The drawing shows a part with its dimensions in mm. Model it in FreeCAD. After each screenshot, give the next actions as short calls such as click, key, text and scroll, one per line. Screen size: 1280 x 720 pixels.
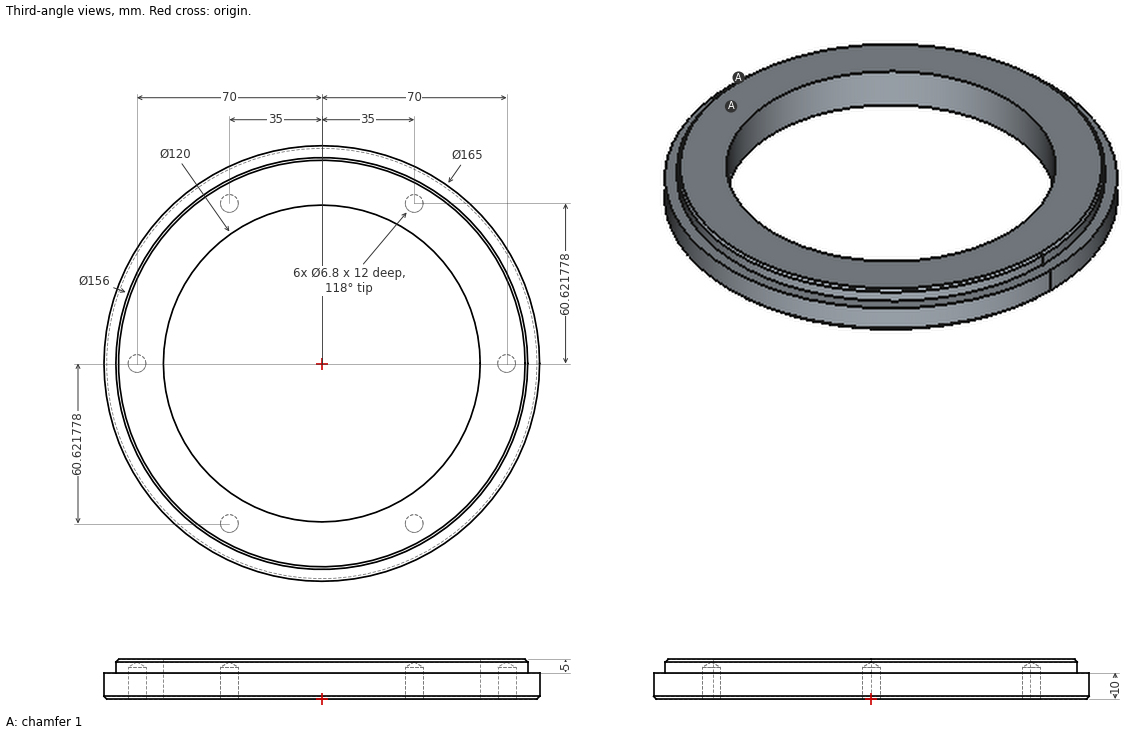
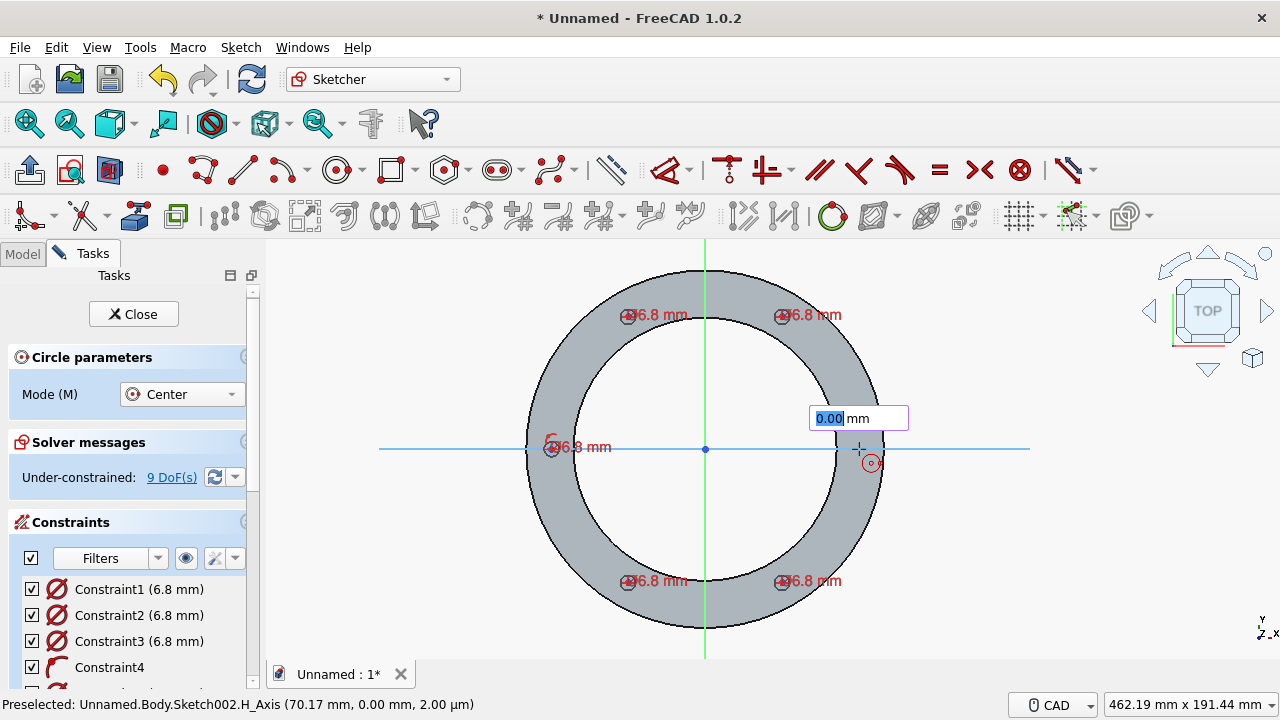
scroll(856, 456, up, 5)
move(855, 456)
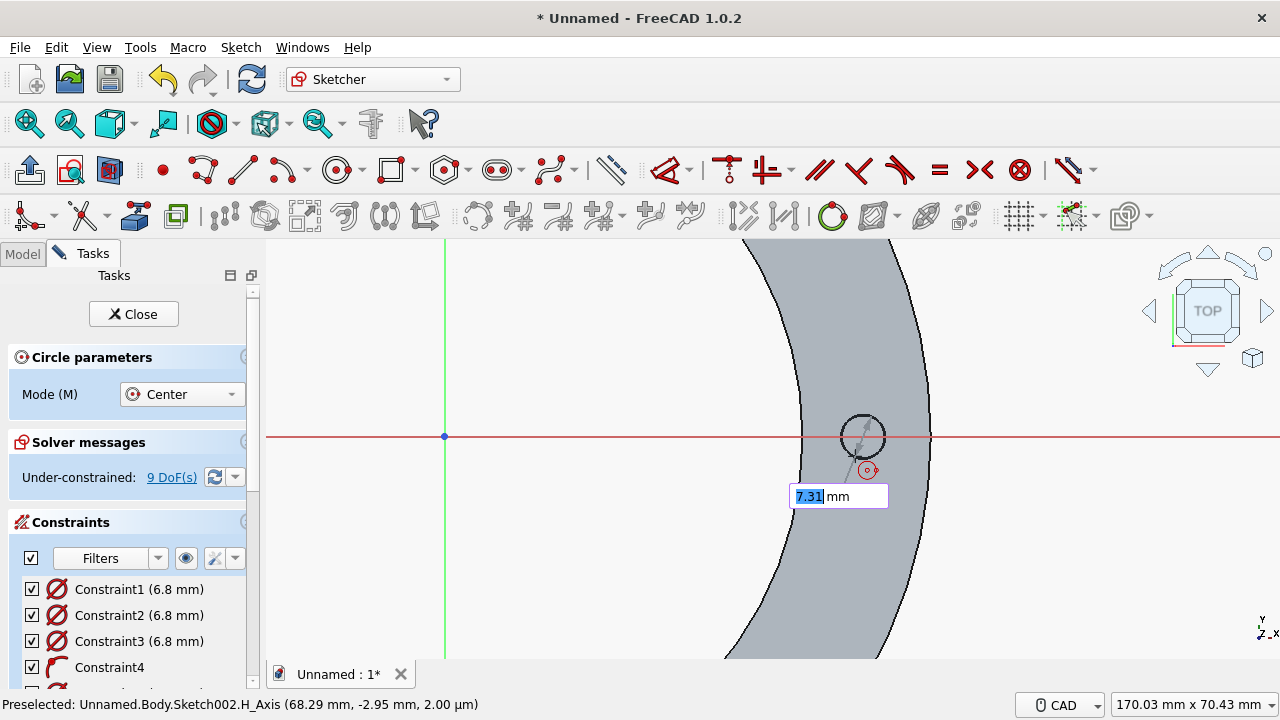
text(6.8)
key(Return)
key(Escape)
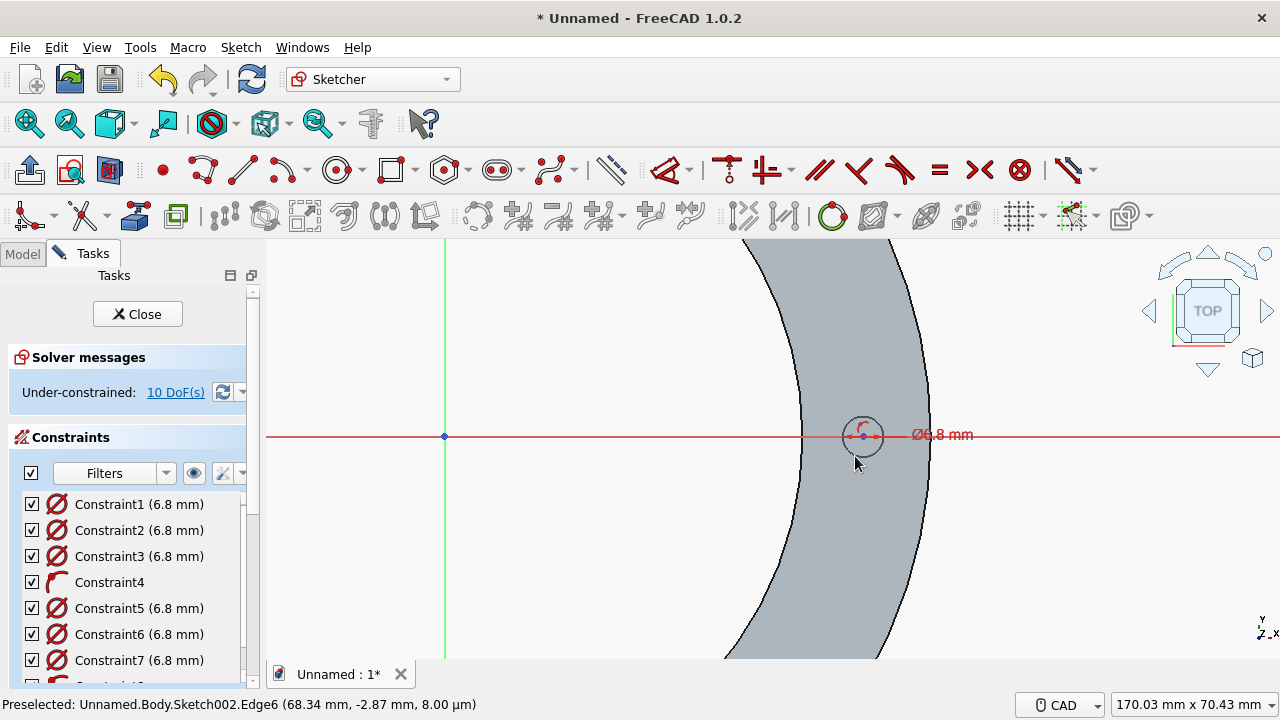
scroll(856, 456, down, 5)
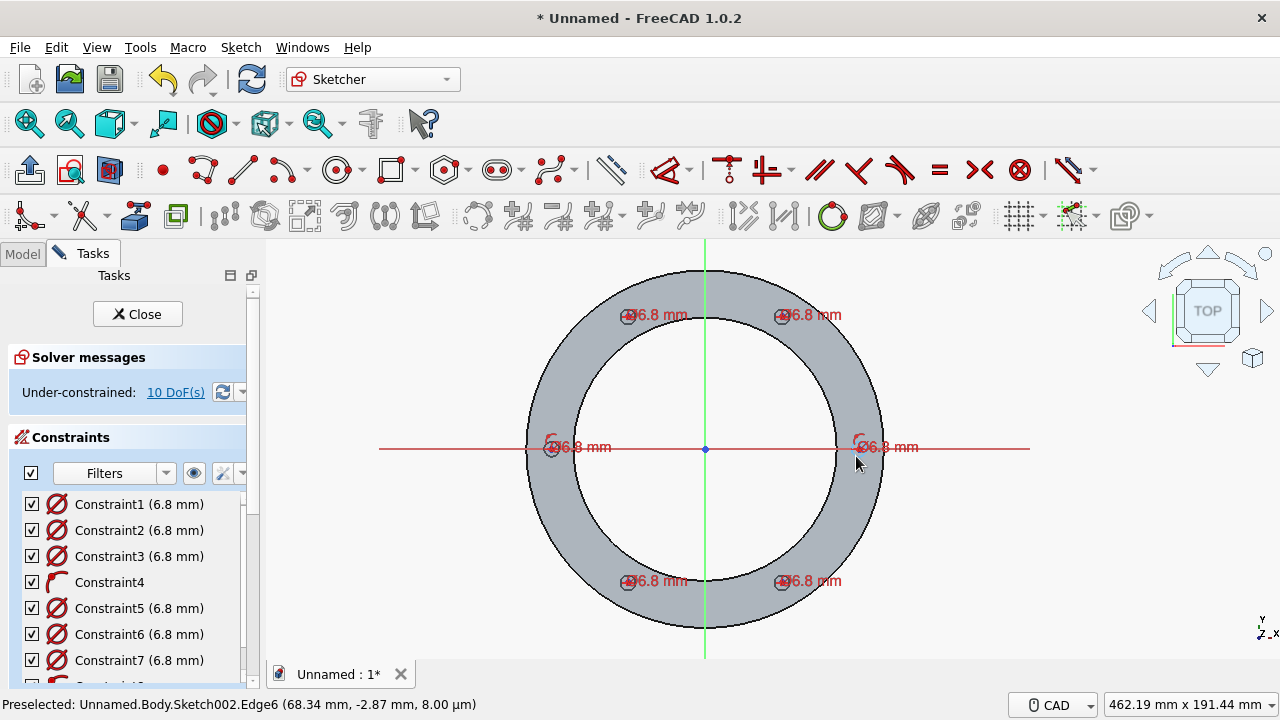
click(782, 317)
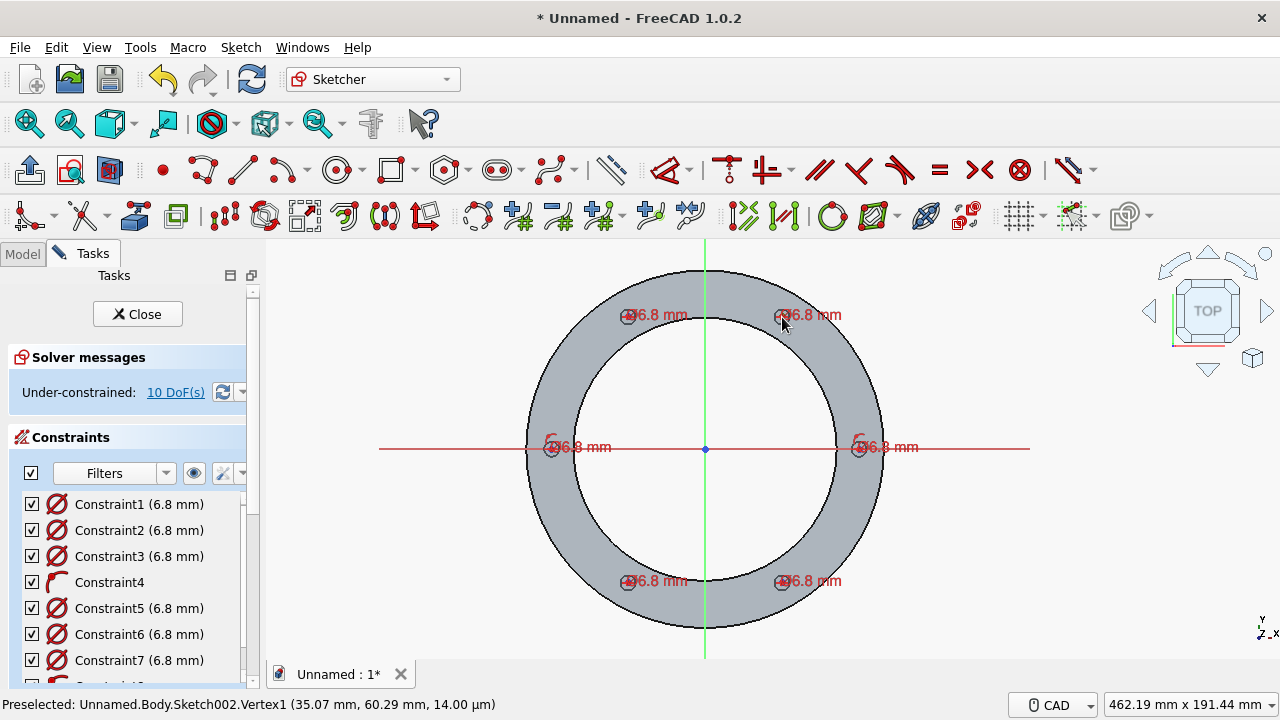
click(628, 317)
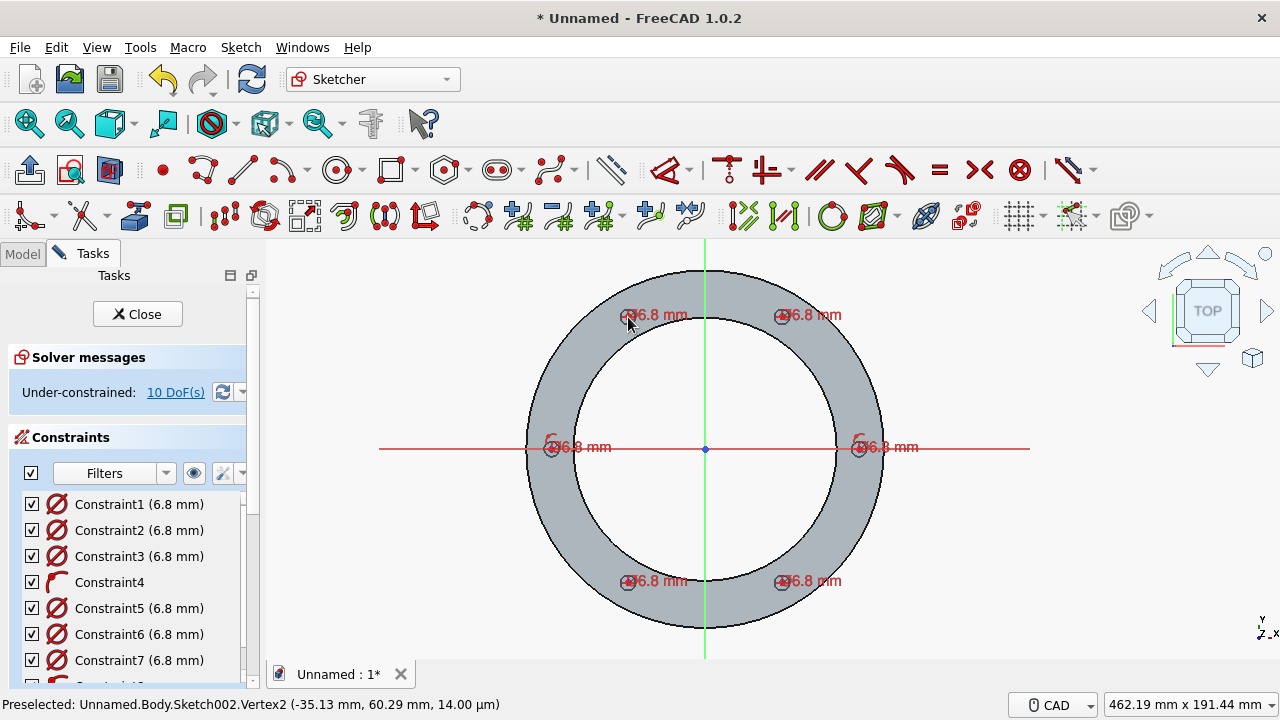
click(794, 170)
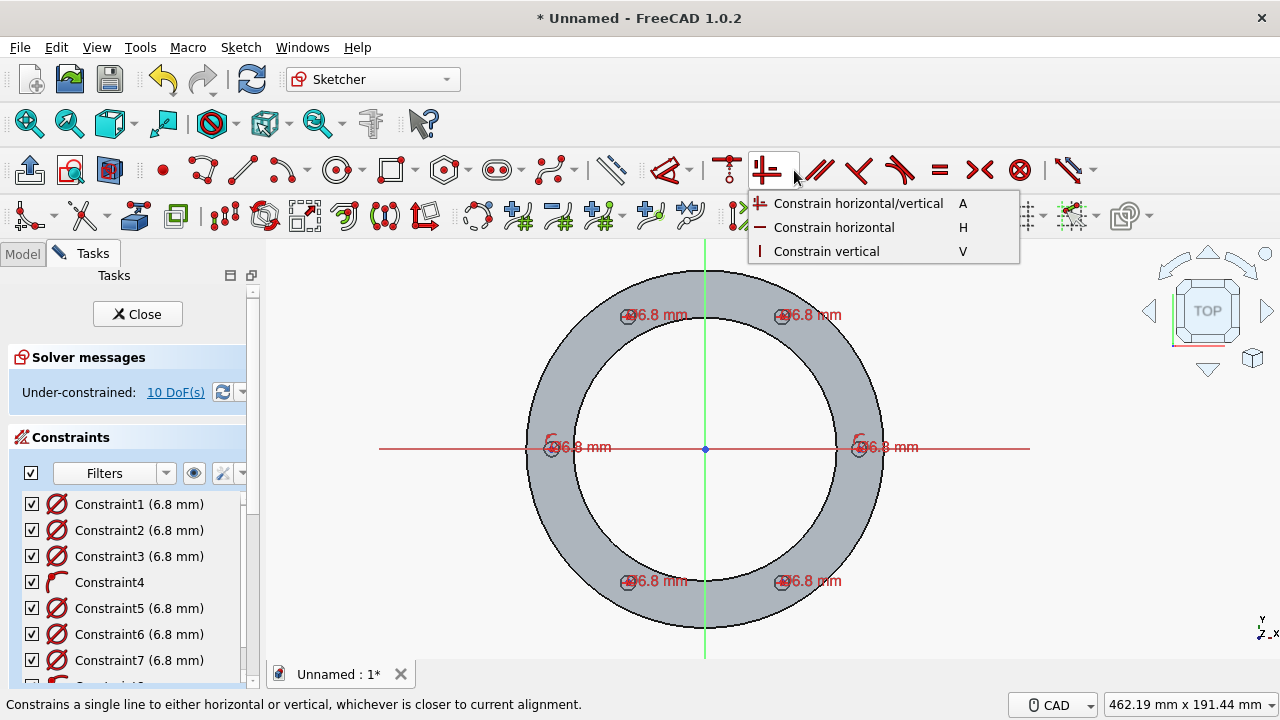
click(884, 227)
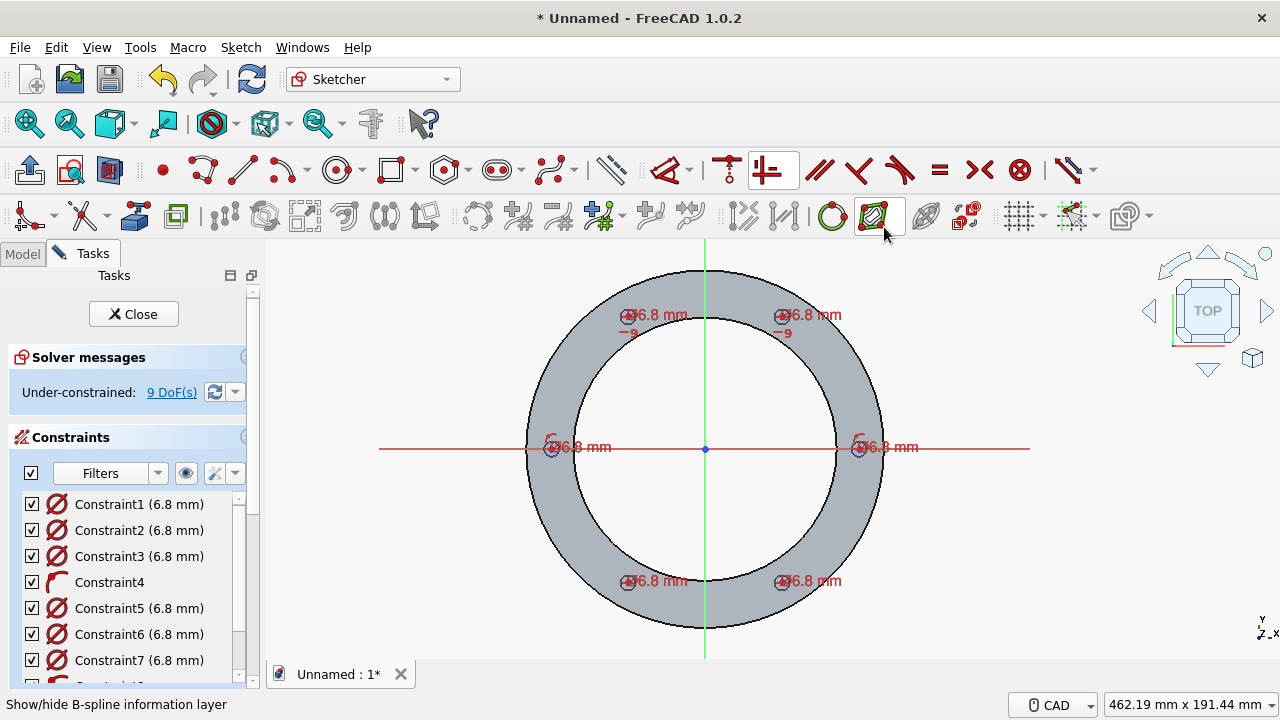
click(628, 317)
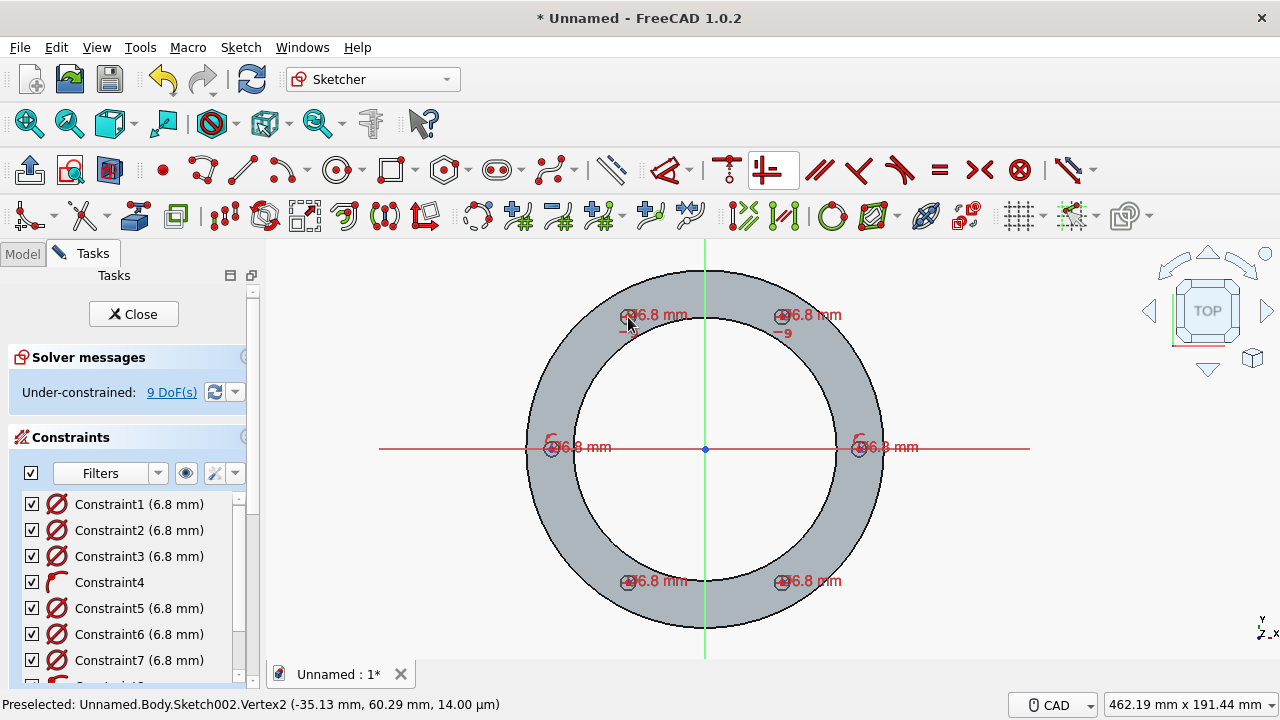
click(628, 583)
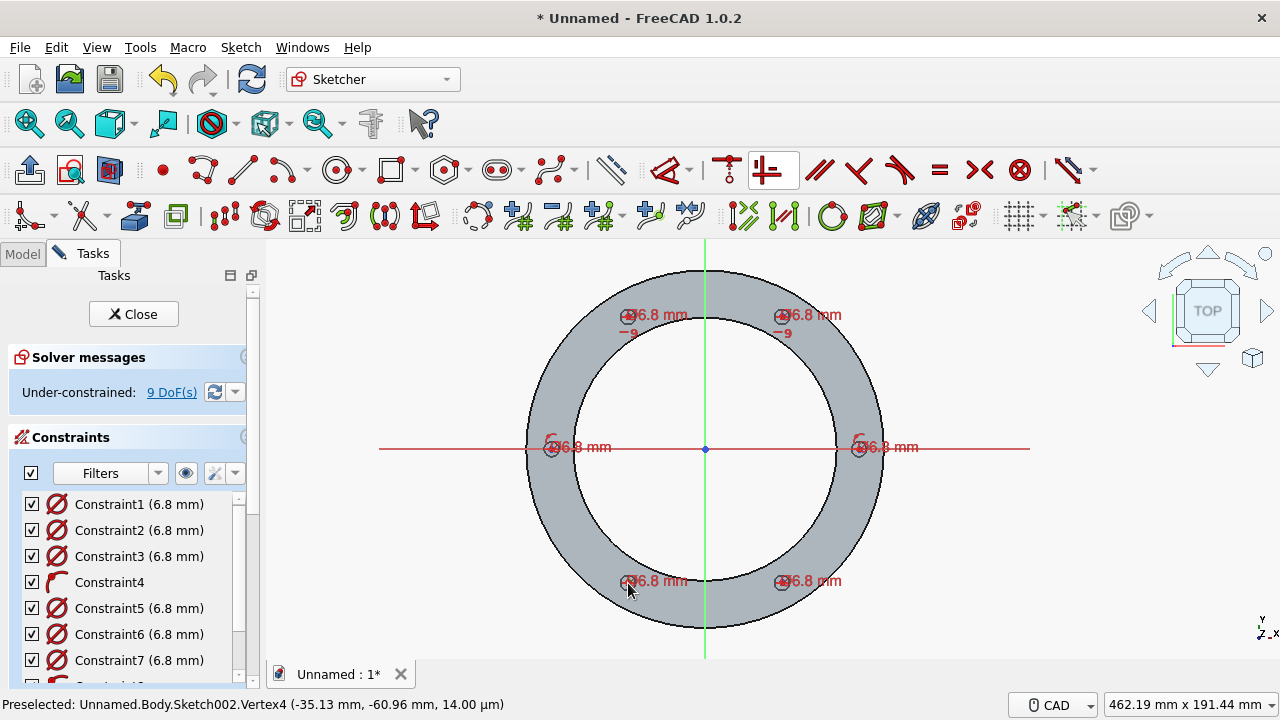
key(v)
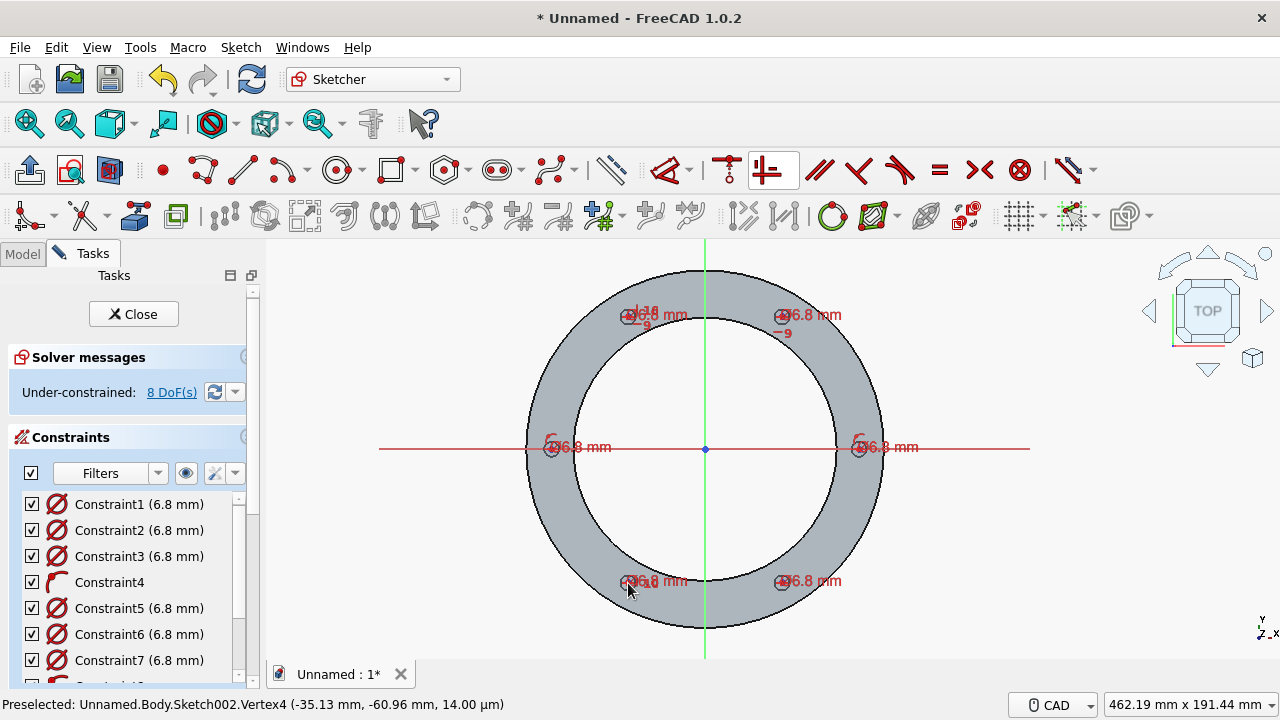
click(782, 317)